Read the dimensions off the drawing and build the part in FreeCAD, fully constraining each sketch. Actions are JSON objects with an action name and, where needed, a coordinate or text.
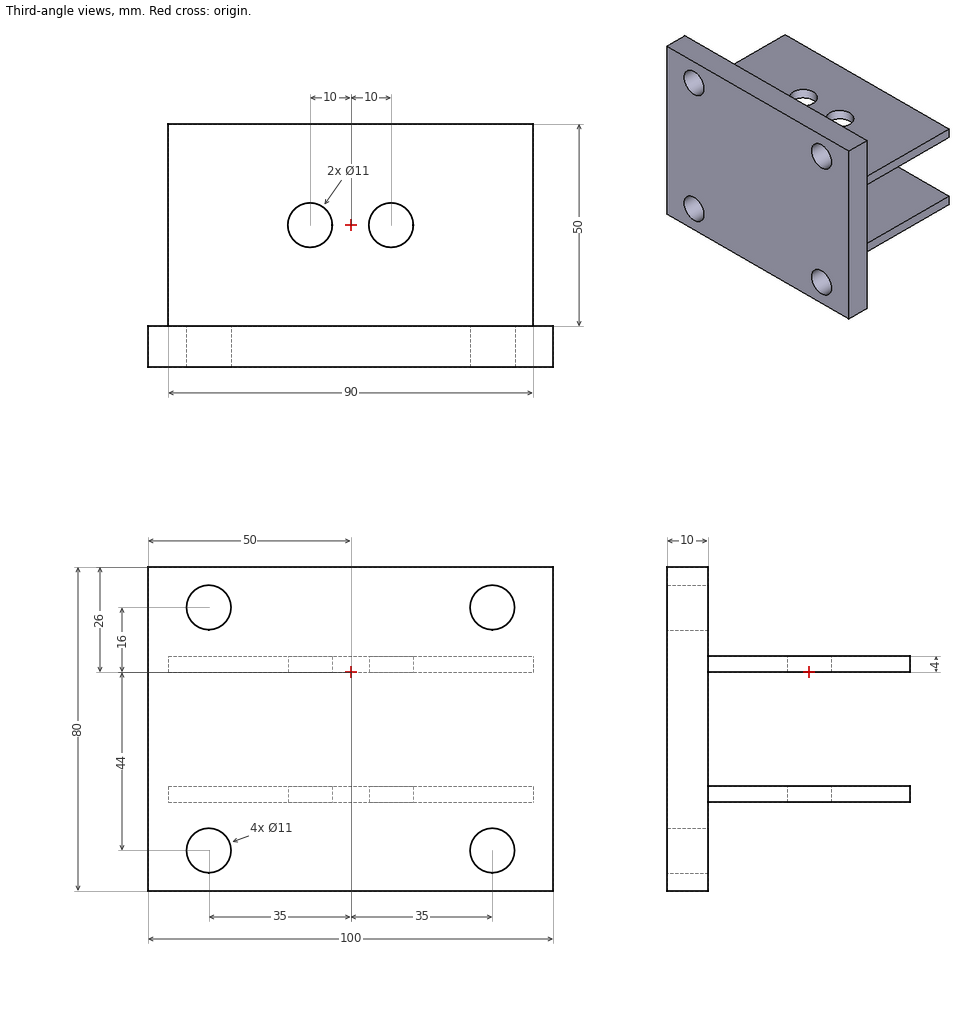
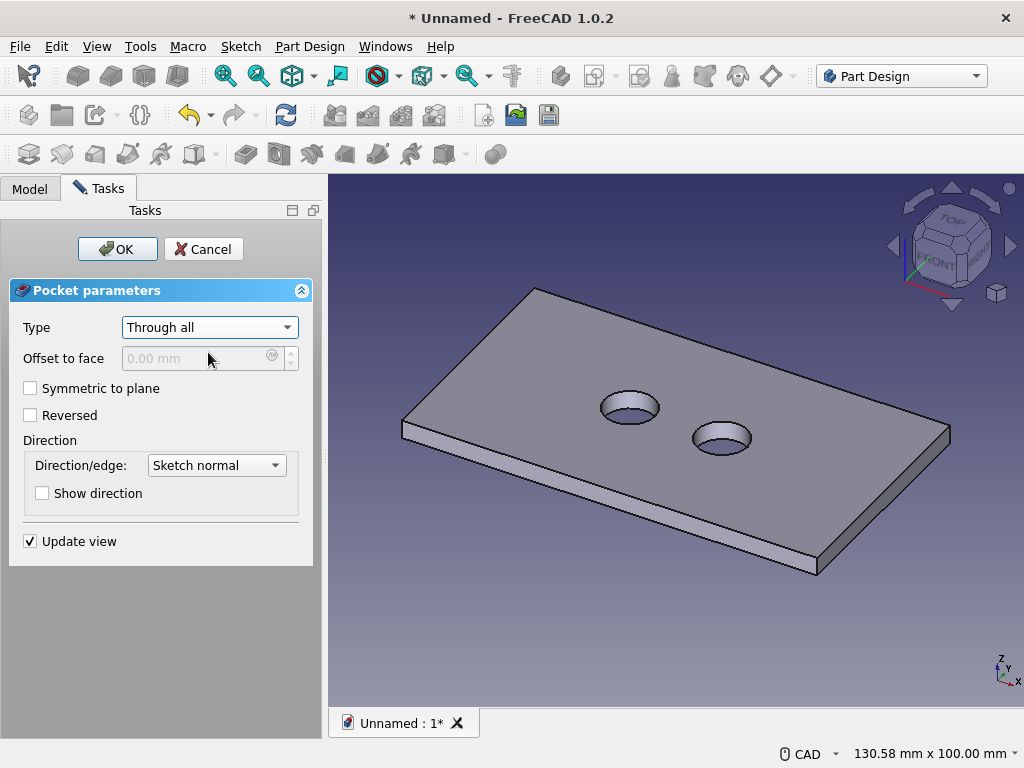
{"action": "left_click", "coordinate": [118, 249]}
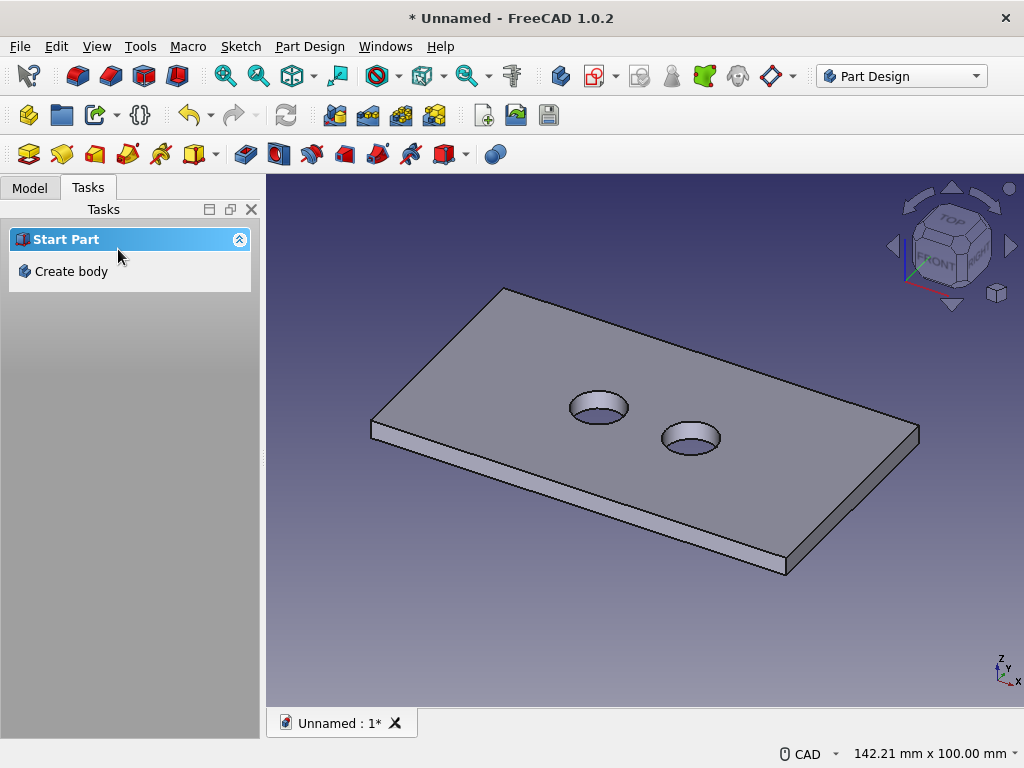
{"action": "key", "text": "0"}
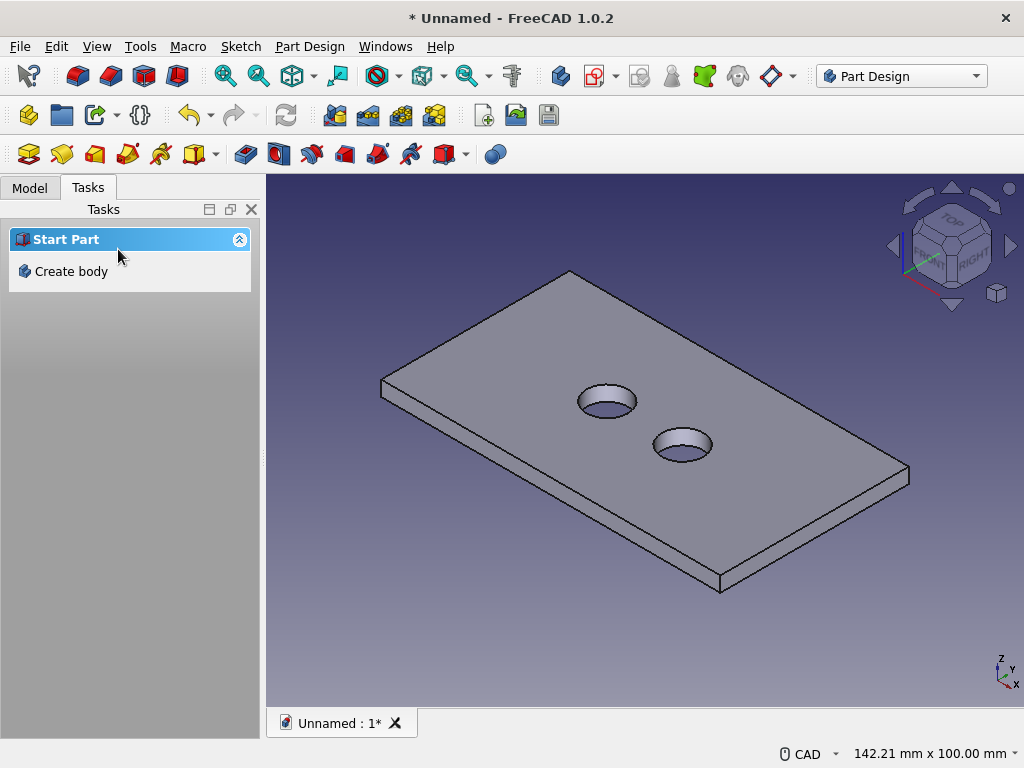
{"action": "key", "text": "1"}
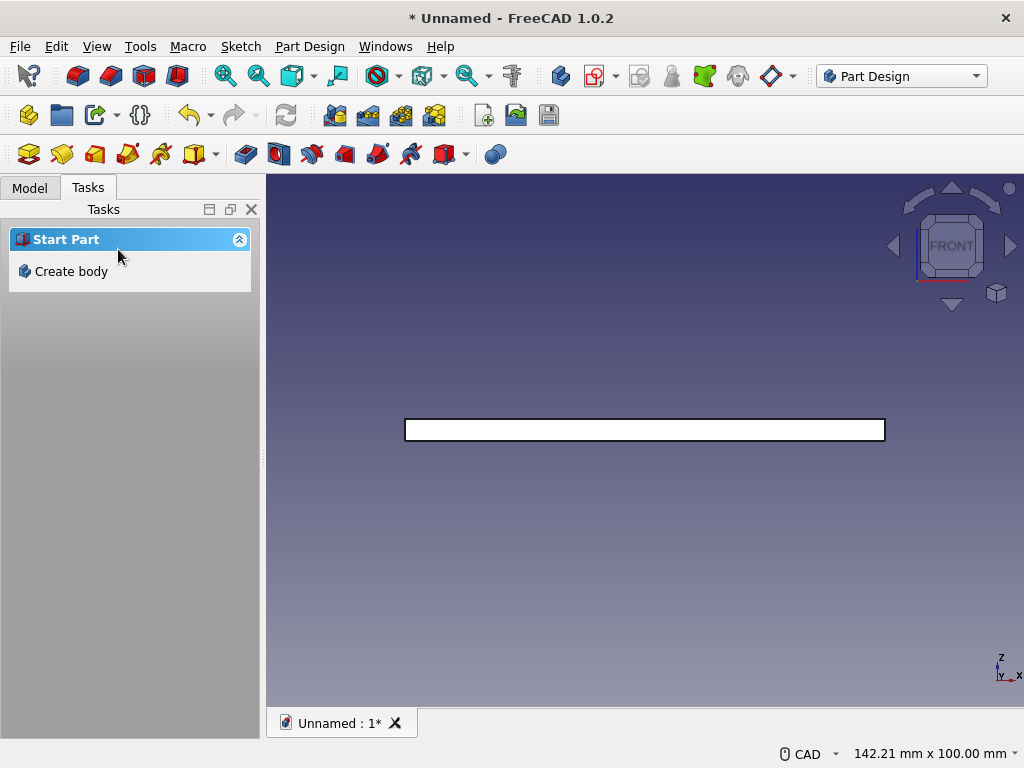
{"action": "left_click", "coordinate": [851, 429]}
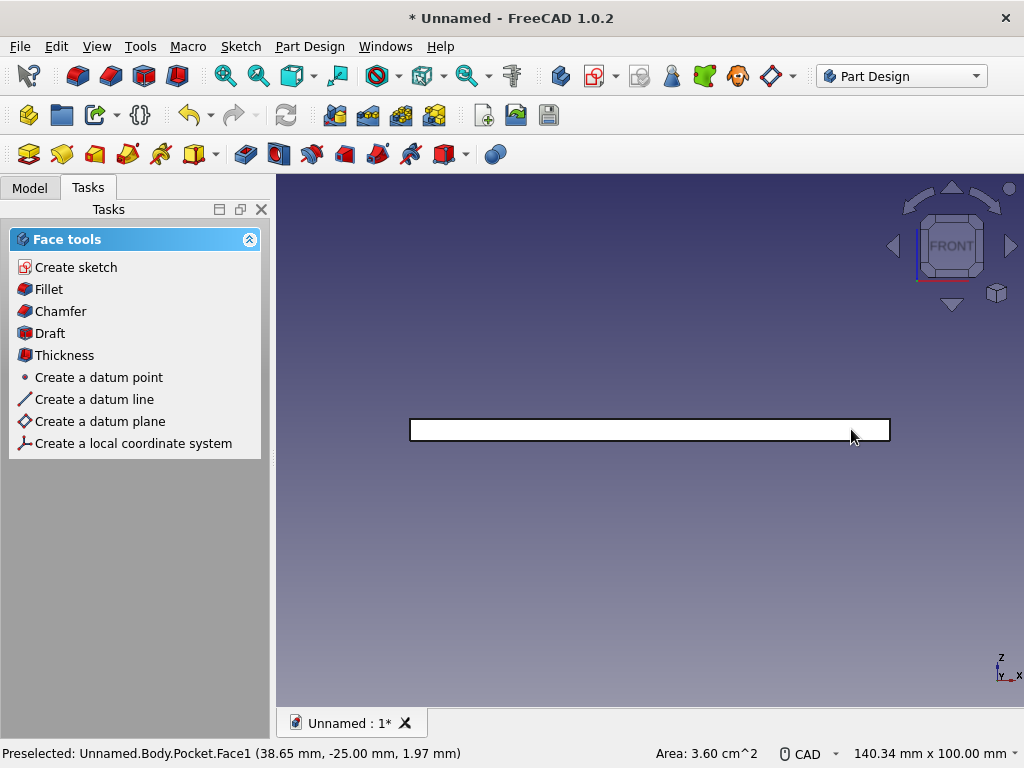
{"action": "left_click", "coordinate": [594, 76]}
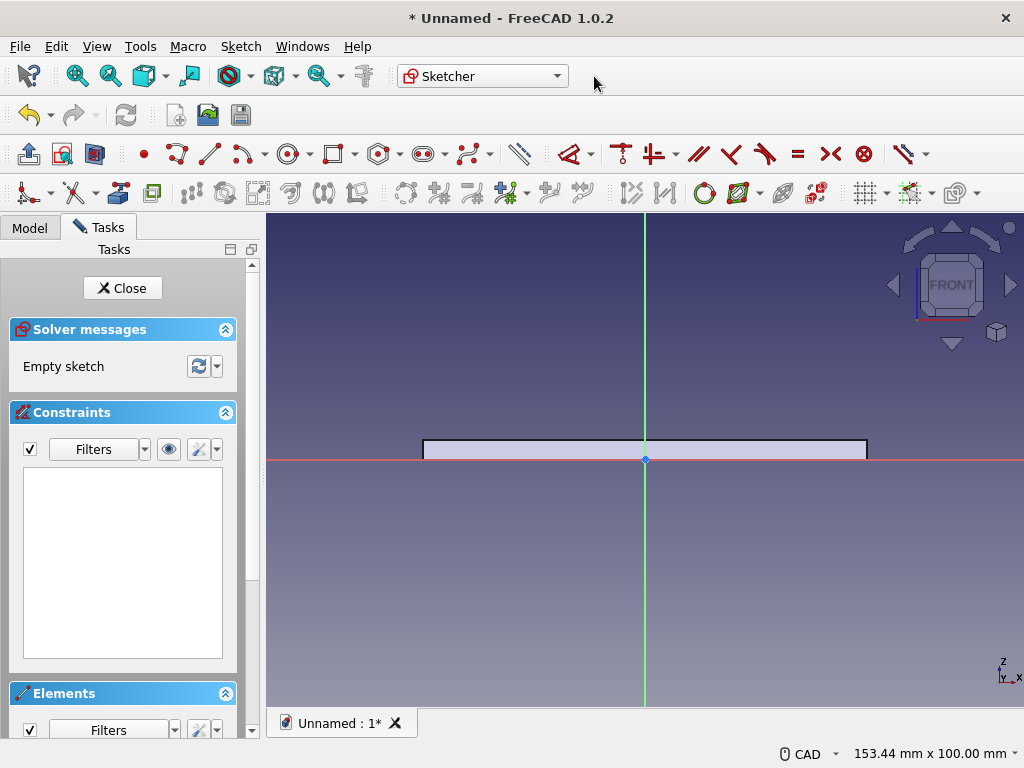
{"action": "scroll", "coordinate": [294, 241], "scroll_direction": "down", "scroll_amount": 1}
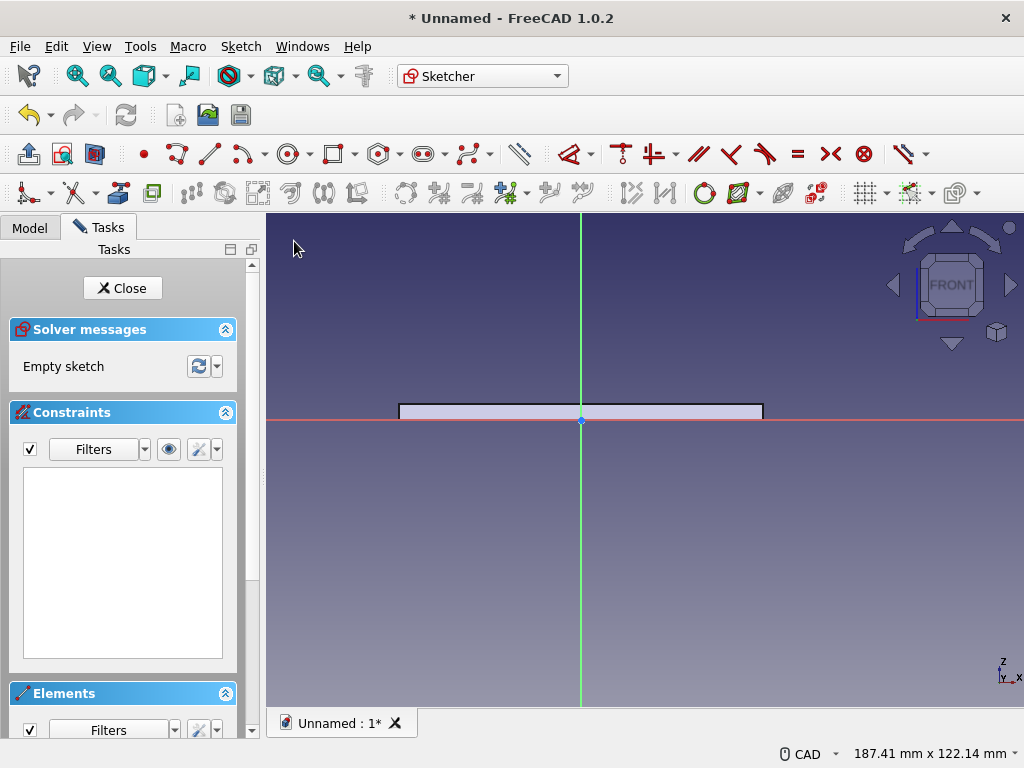
{"action": "key", "text": "g r"}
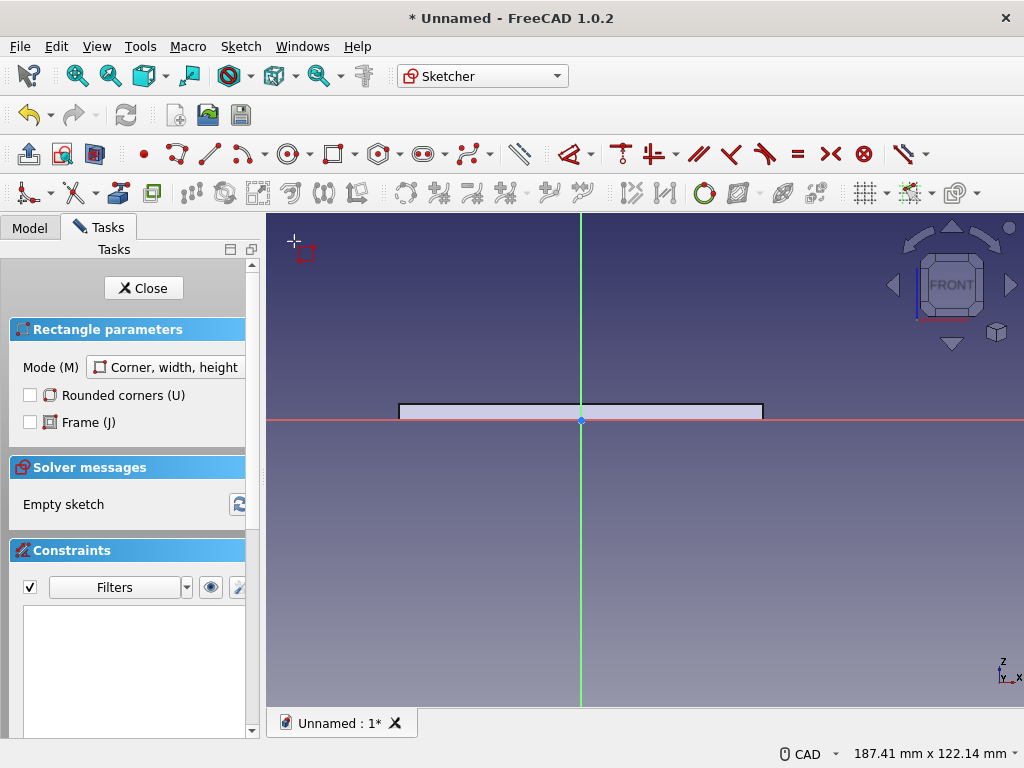
{"action": "left_click", "coordinate": [379, 315]}
{"action": "left_click", "coordinate": [784, 639]}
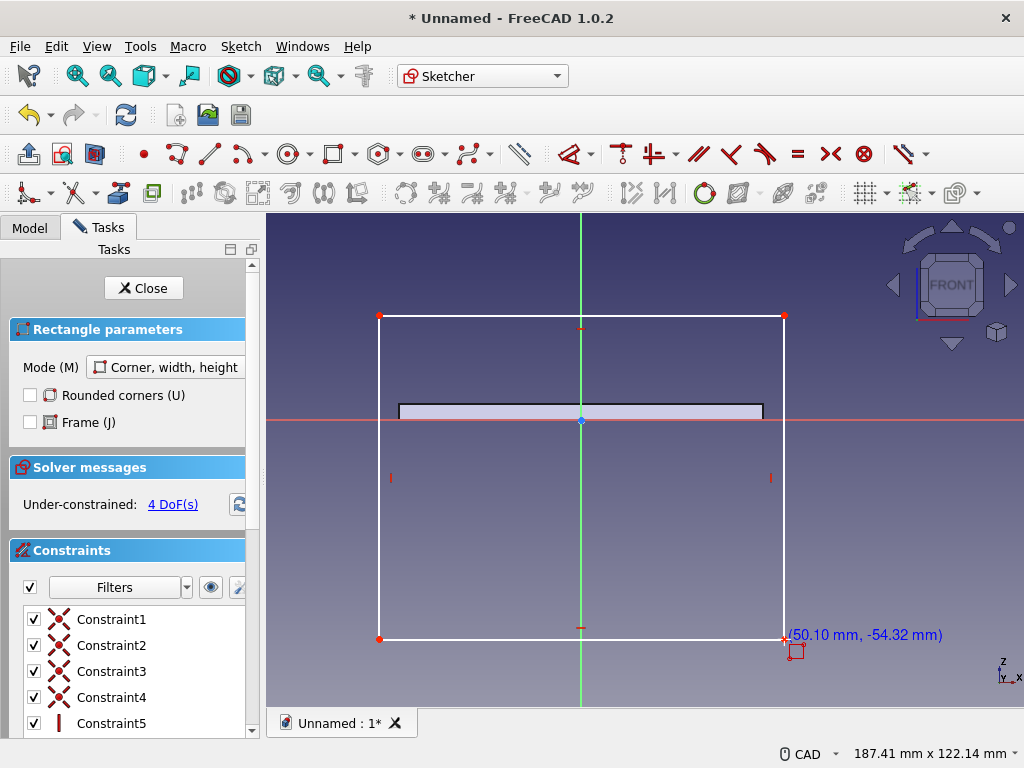
{"action": "left_click", "coordinate": [288, 154]}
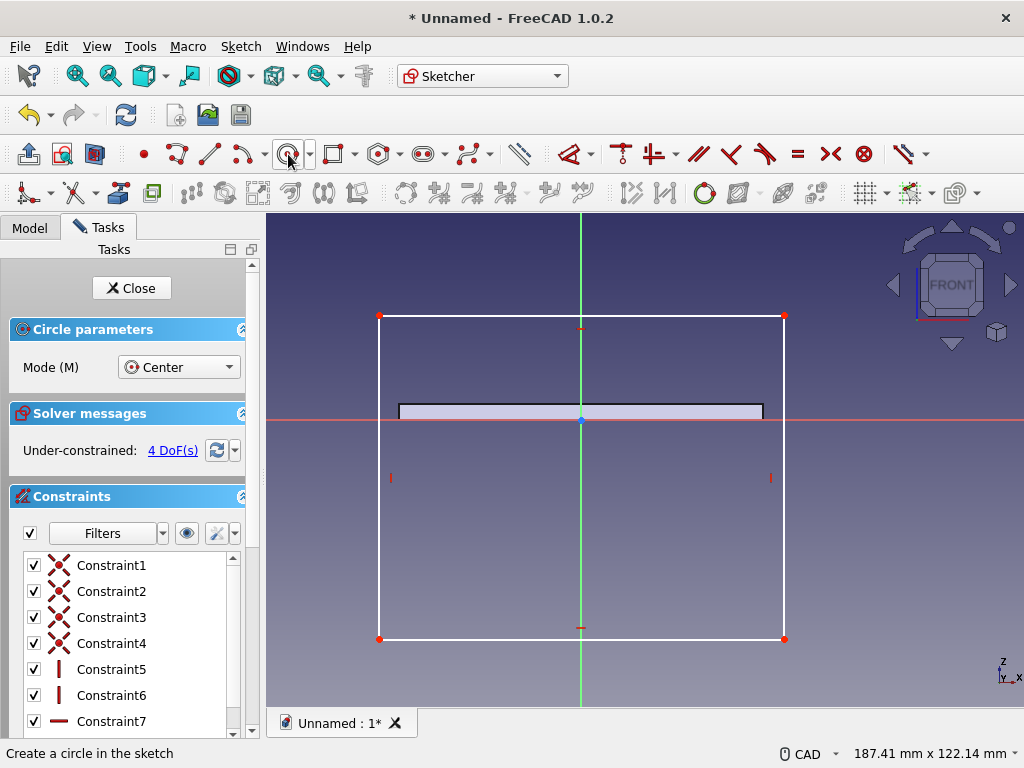
{"action": "left_click", "coordinate": [440, 598]}
{"action": "left_click", "coordinate": [456, 583]}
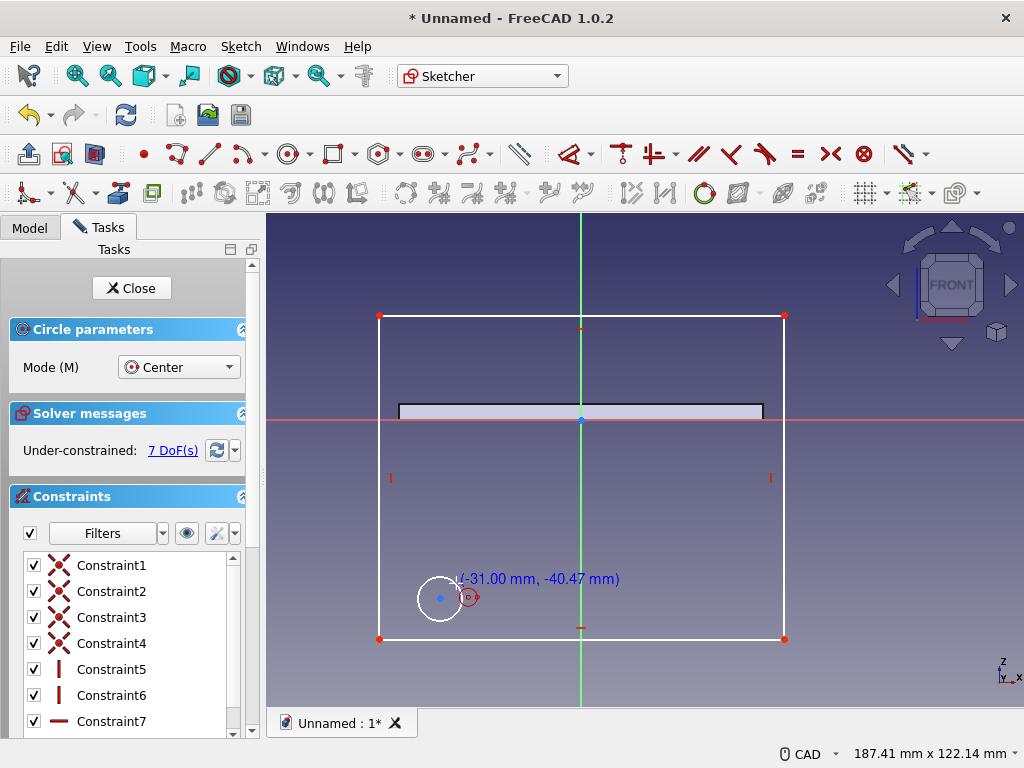
{"action": "left_click", "coordinate": [723, 598]}
{"action": "left_click", "coordinate": [739, 583]}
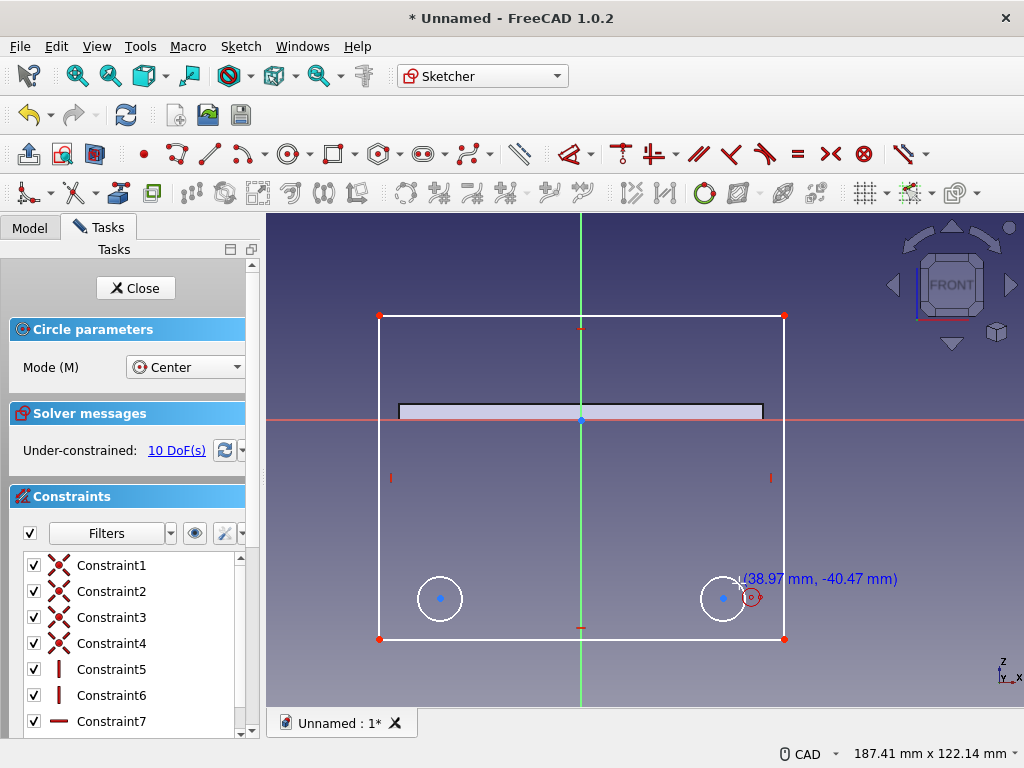
{"action": "left_click", "coordinate": [440, 356]}
{"action": "left_click", "coordinate": [456, 340]}